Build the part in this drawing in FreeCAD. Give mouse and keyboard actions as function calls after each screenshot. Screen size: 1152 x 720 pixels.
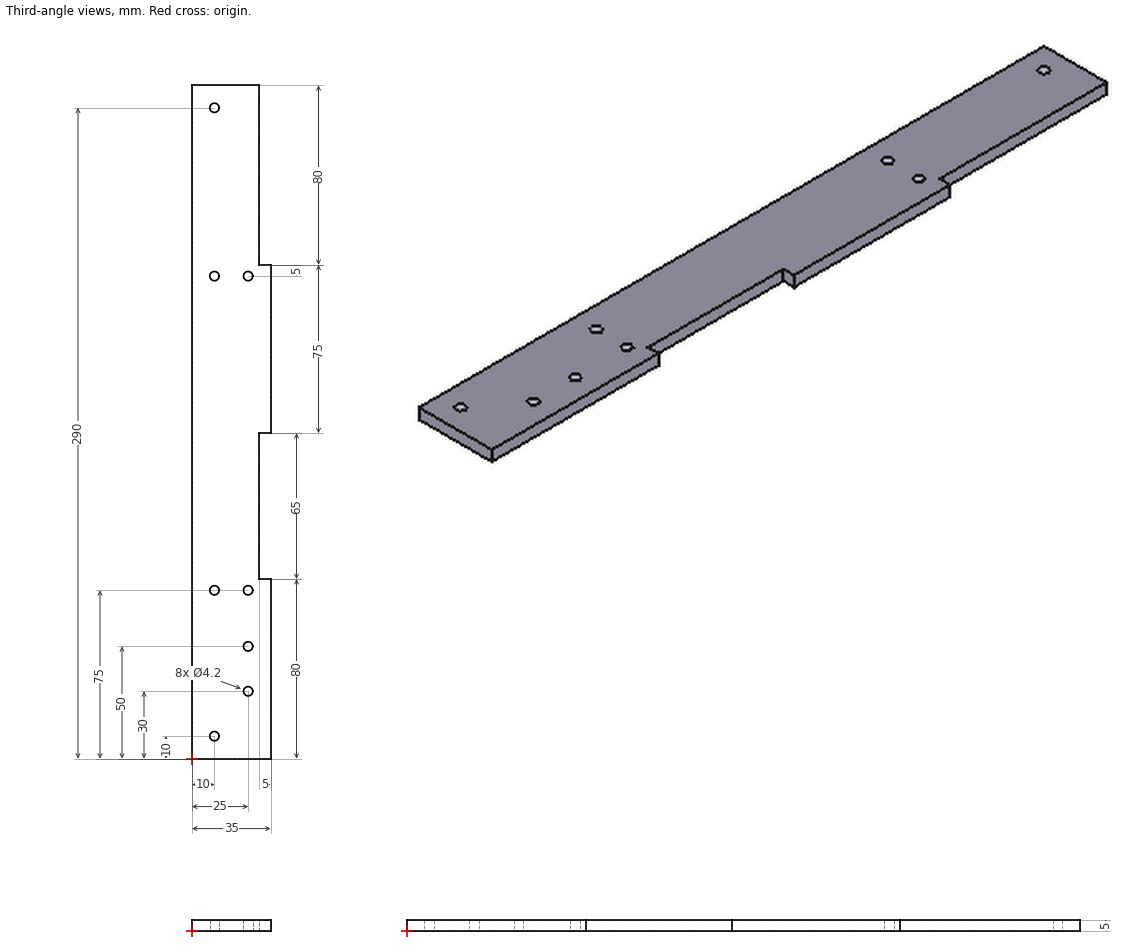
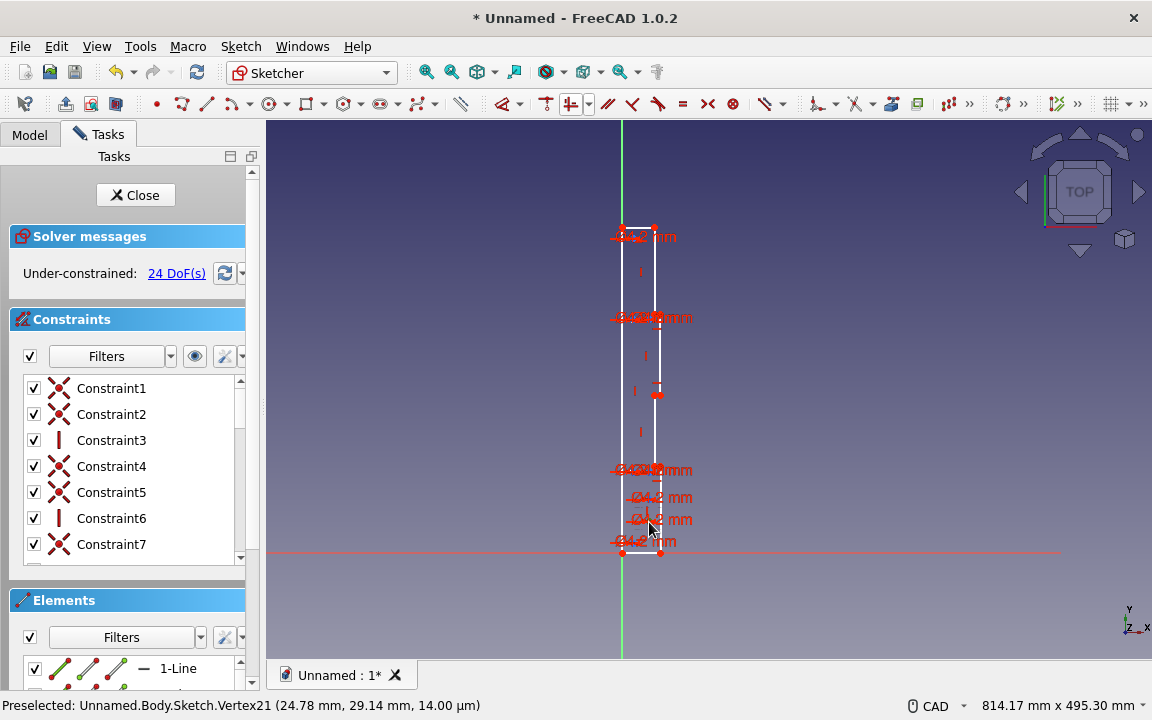
click(649, 500)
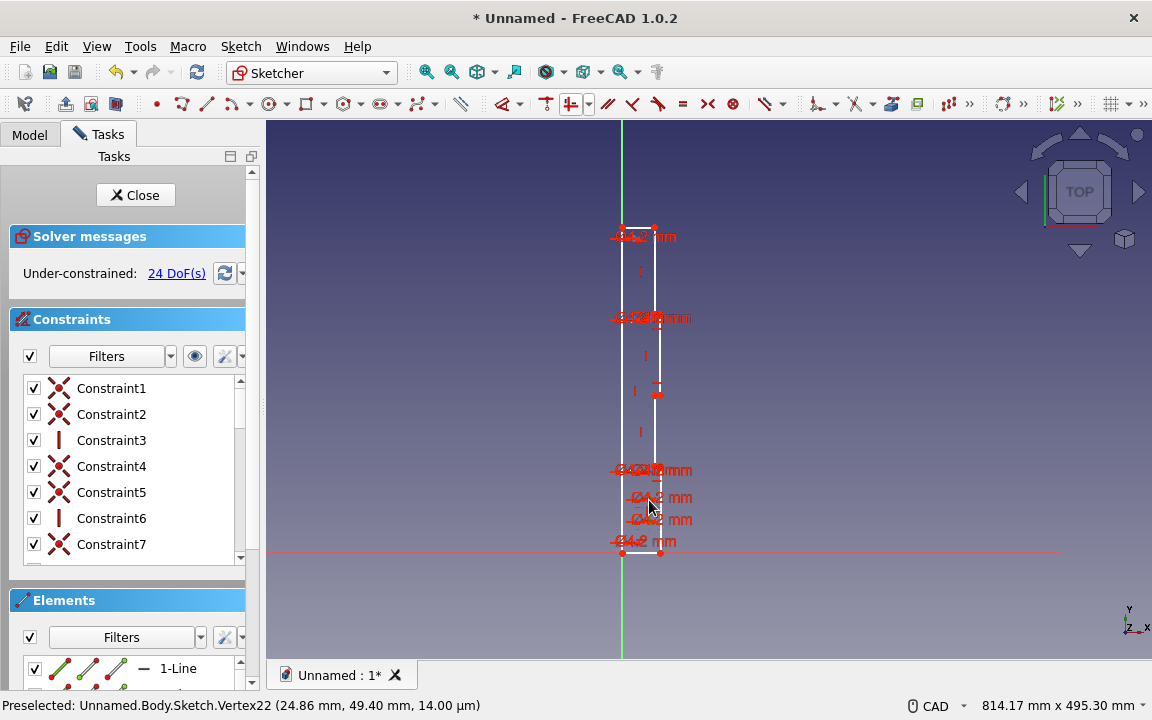
click(588, 104)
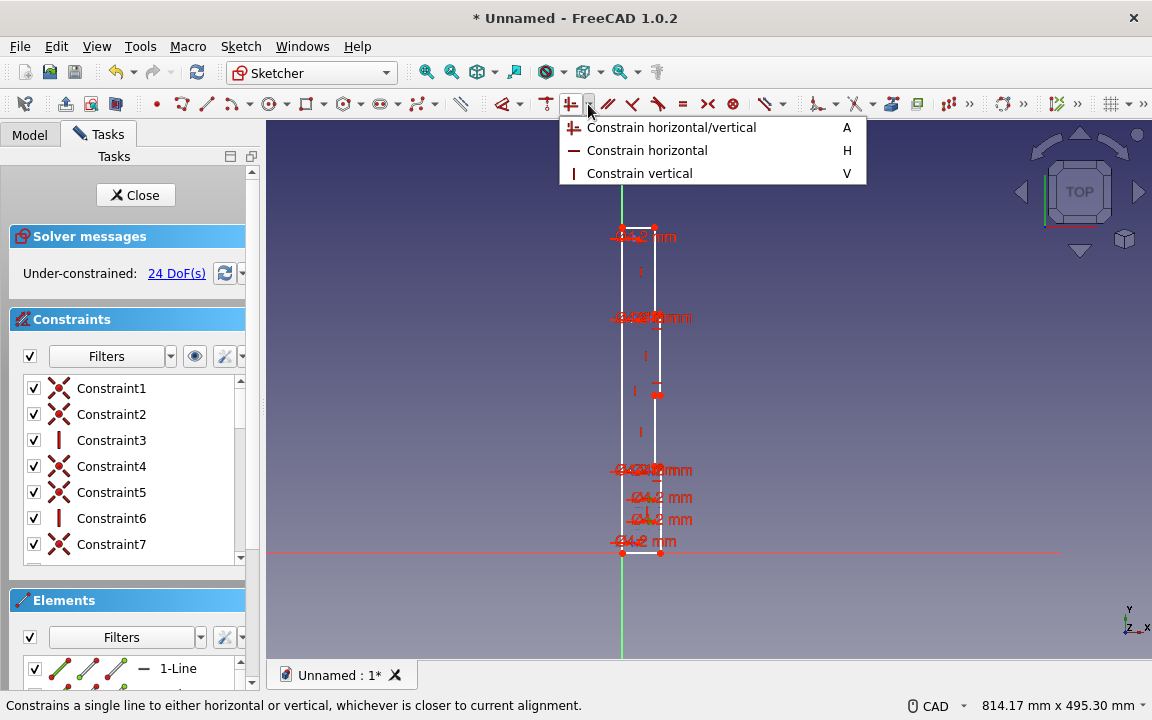
click(713, 174)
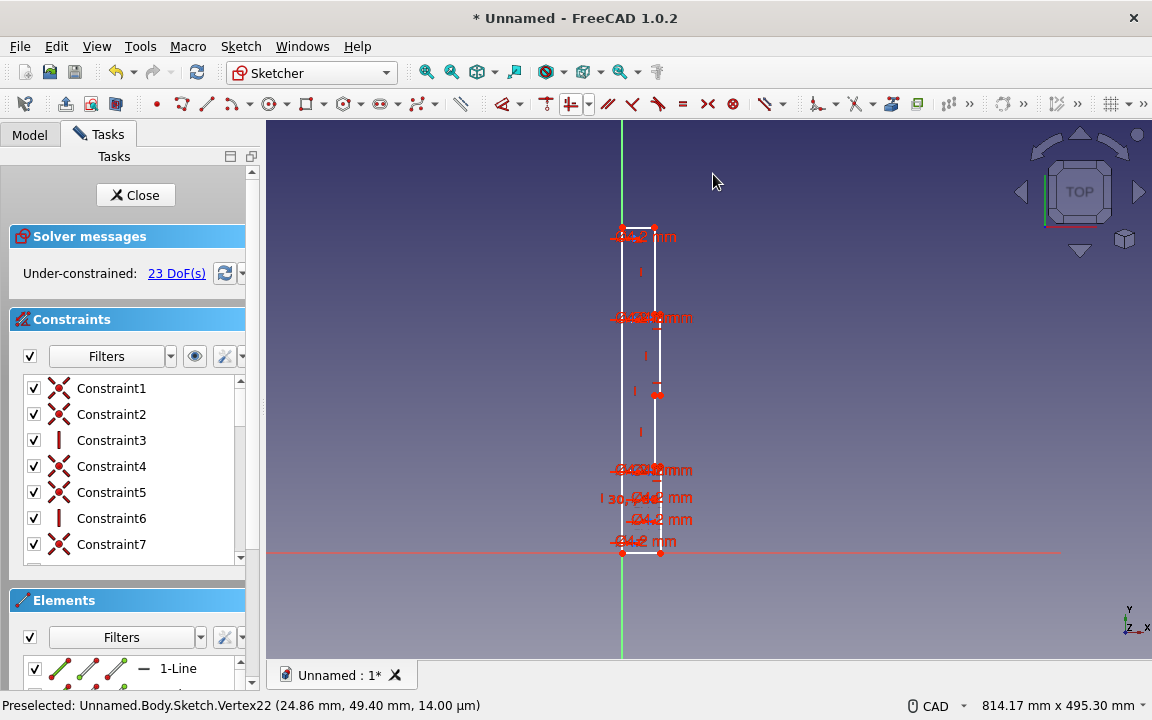
scroll(649, 500, up, 4)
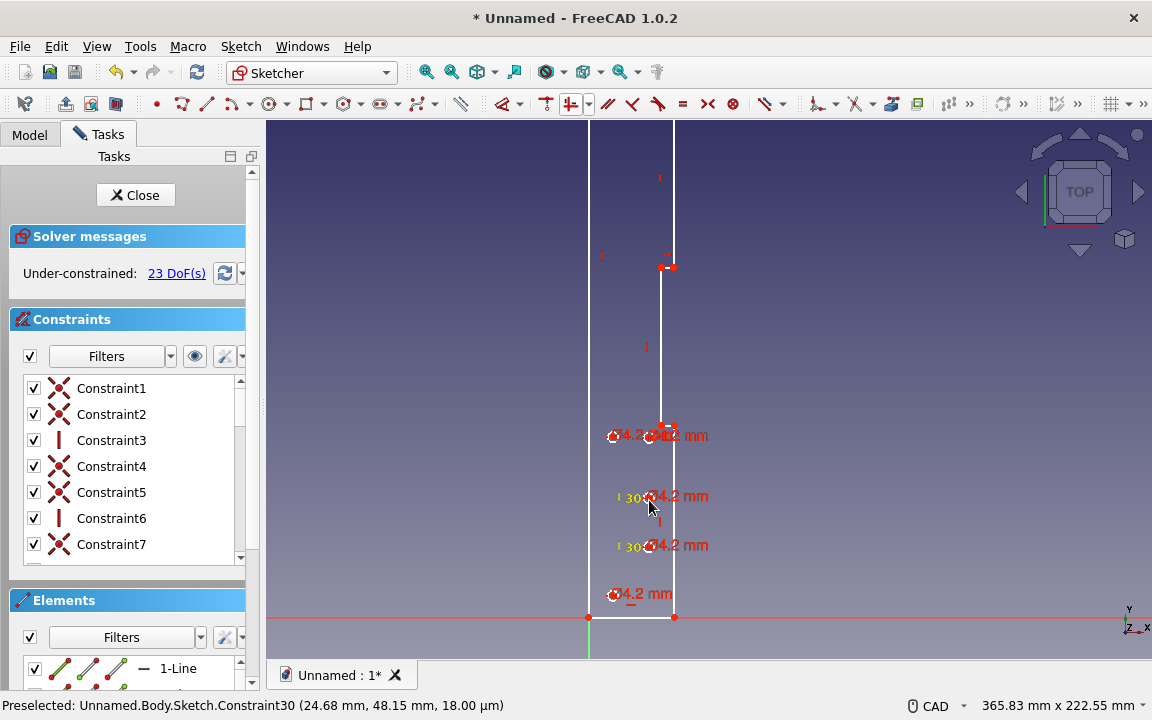
click(649, 498)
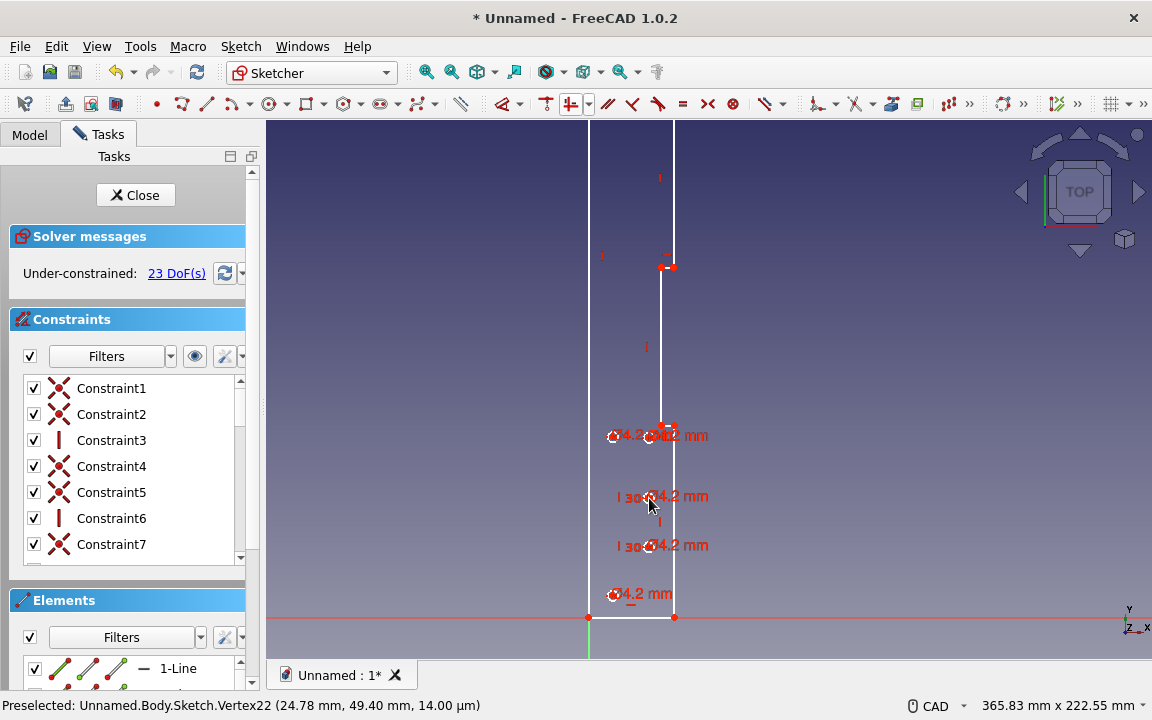
click(649, 438)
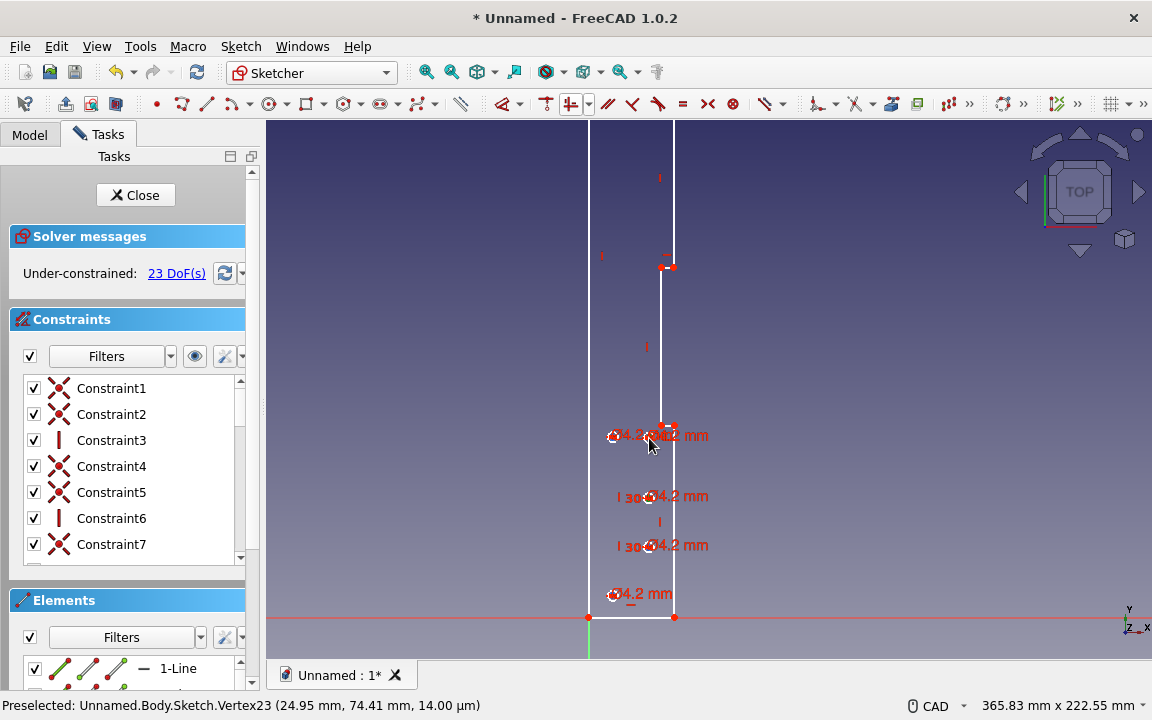
key(v)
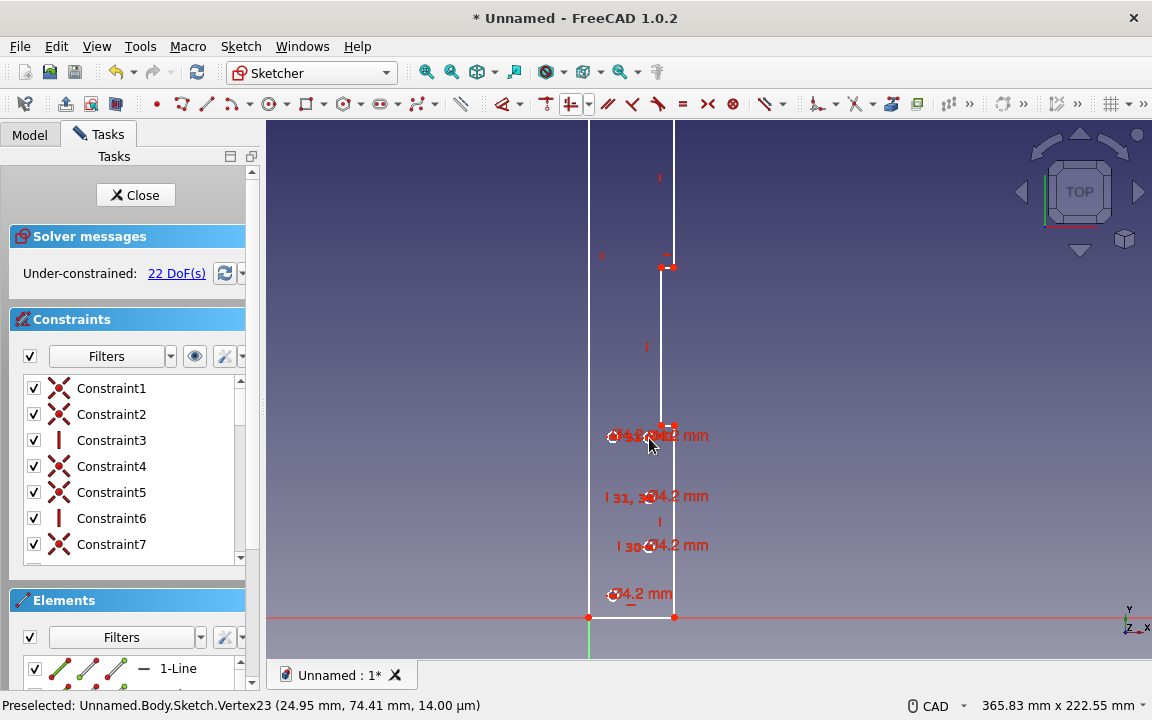
click(649, 438)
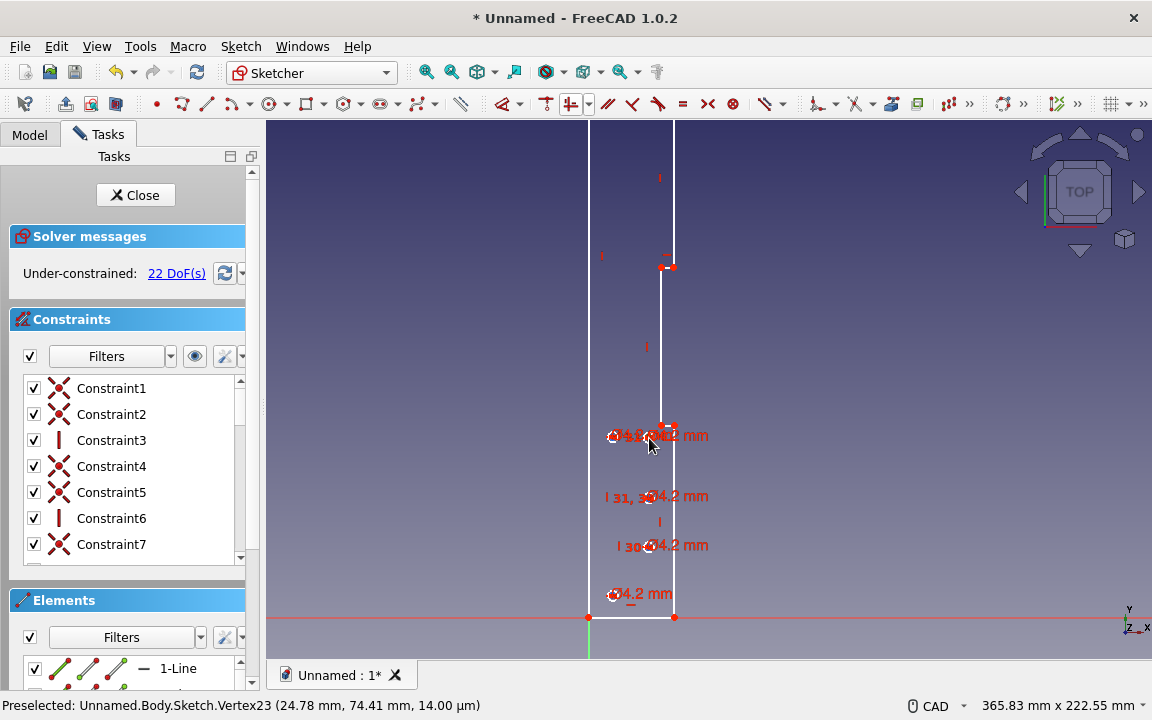
click(613, 437)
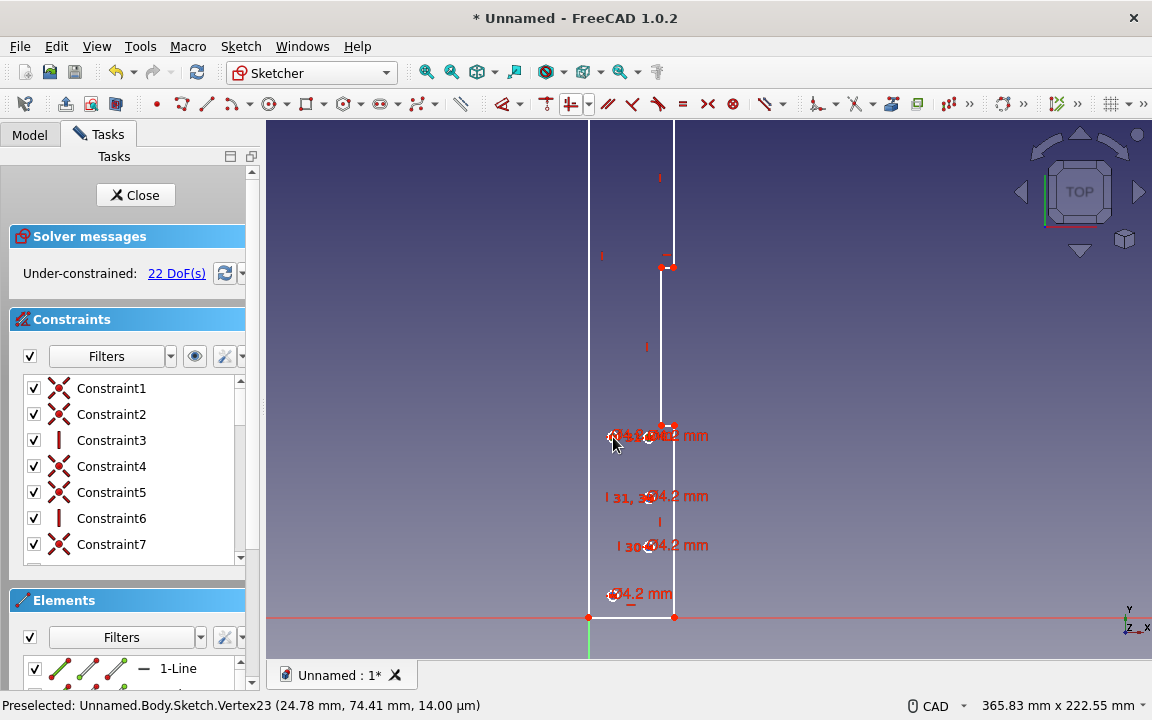
key(h)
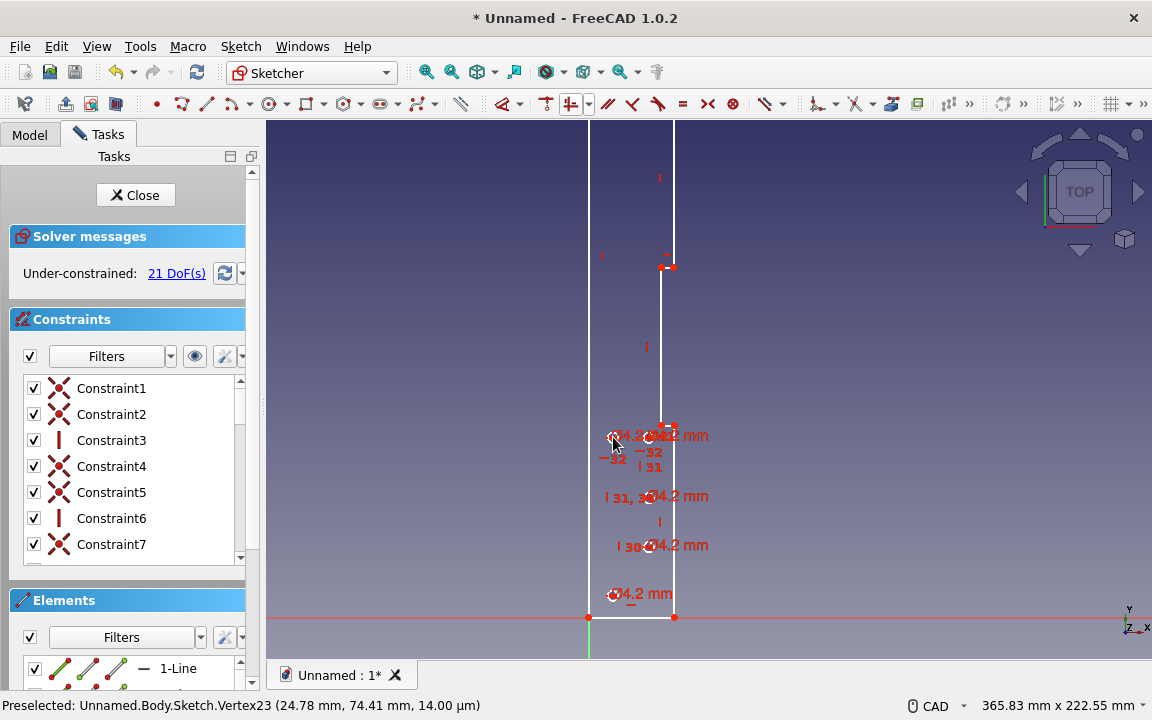
scroll(648, 500, down, 4)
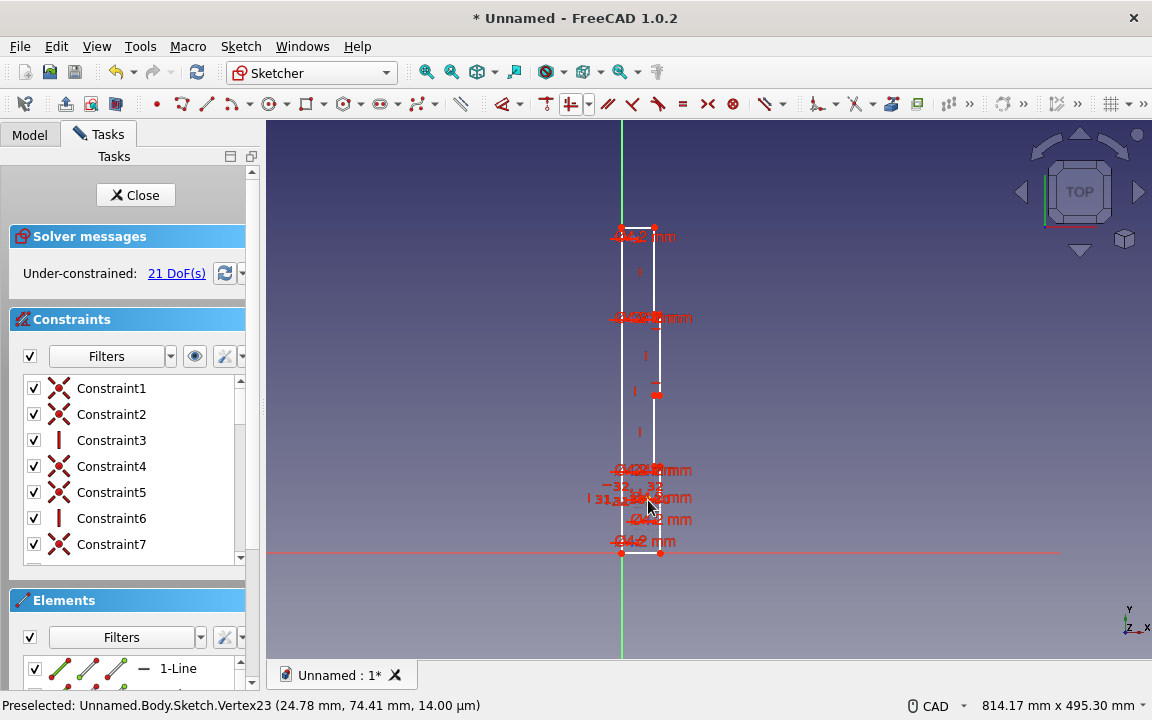
scroll(649, 320, up, 3)